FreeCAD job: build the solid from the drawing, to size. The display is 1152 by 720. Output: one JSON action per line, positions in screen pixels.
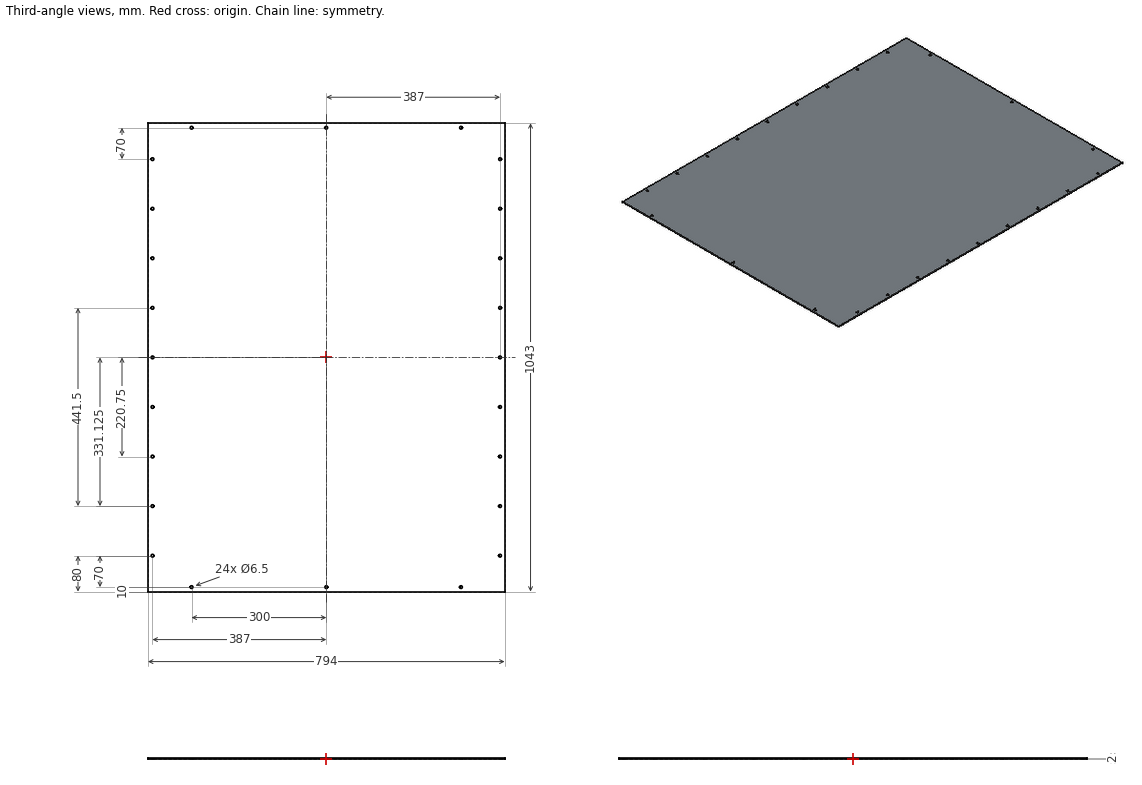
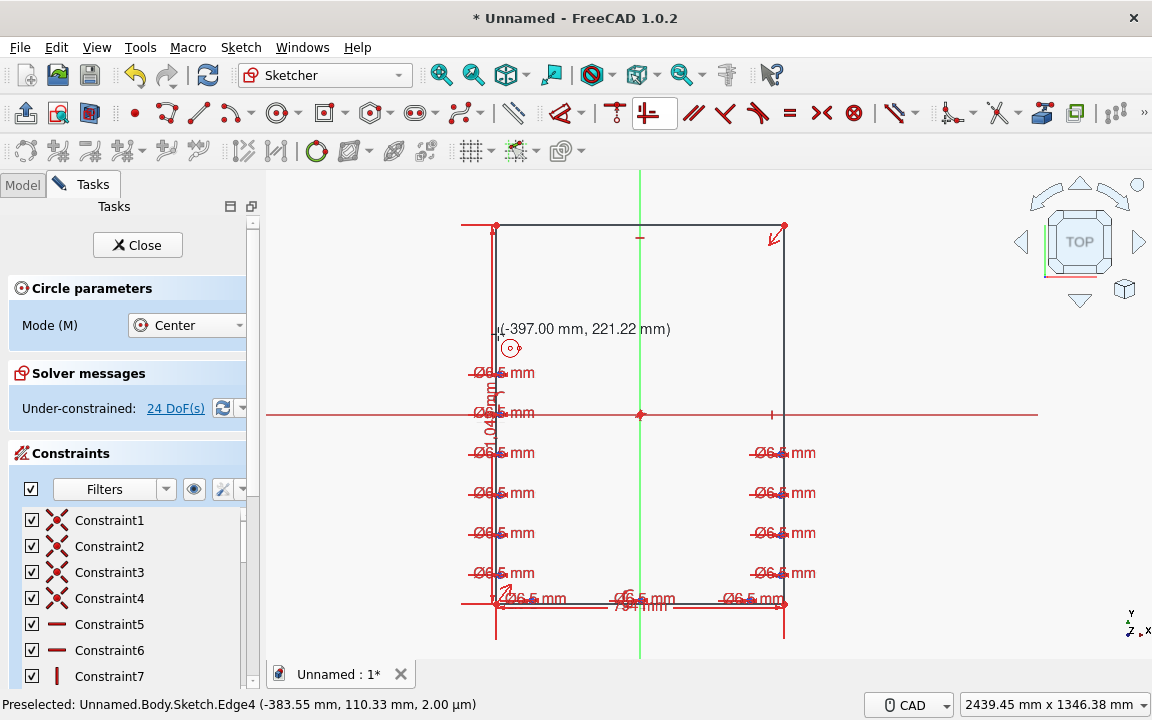
{"action": "scroll", "coordinate": [500, 335], "scroll_direction": "up", "scroll_amount": 8}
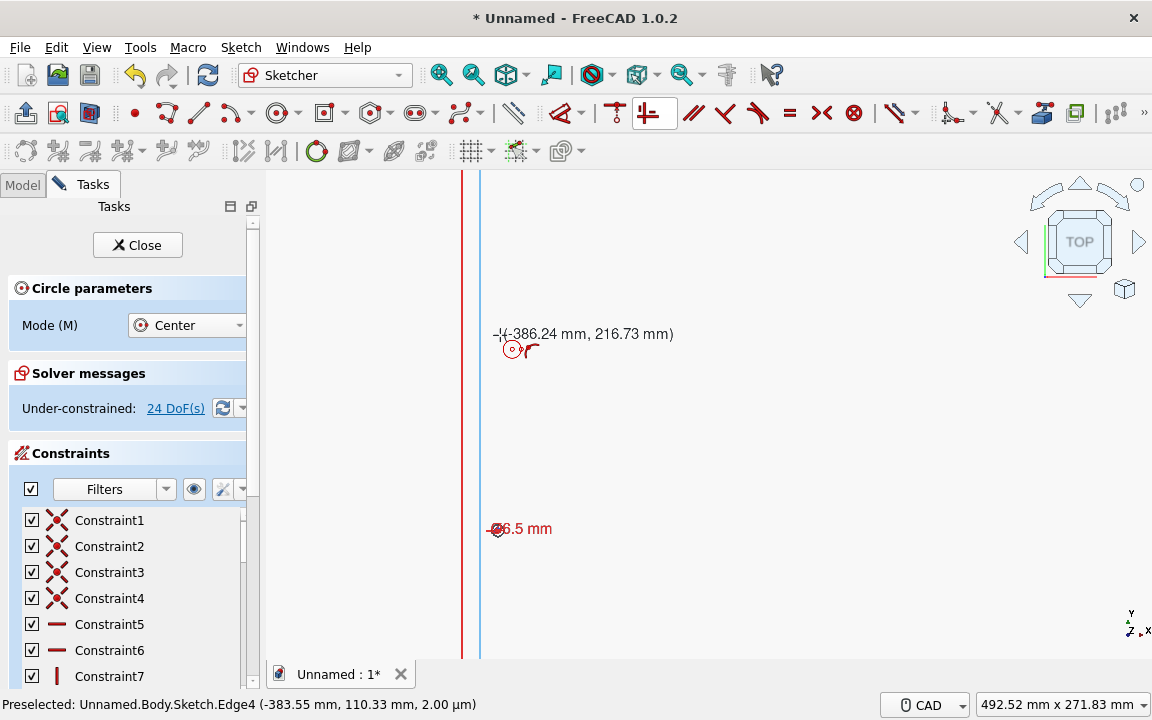
{"action": "left_click", "coordinate": [498, 331]}
{"action": "mouse_move", "coordinate": [502, 327]}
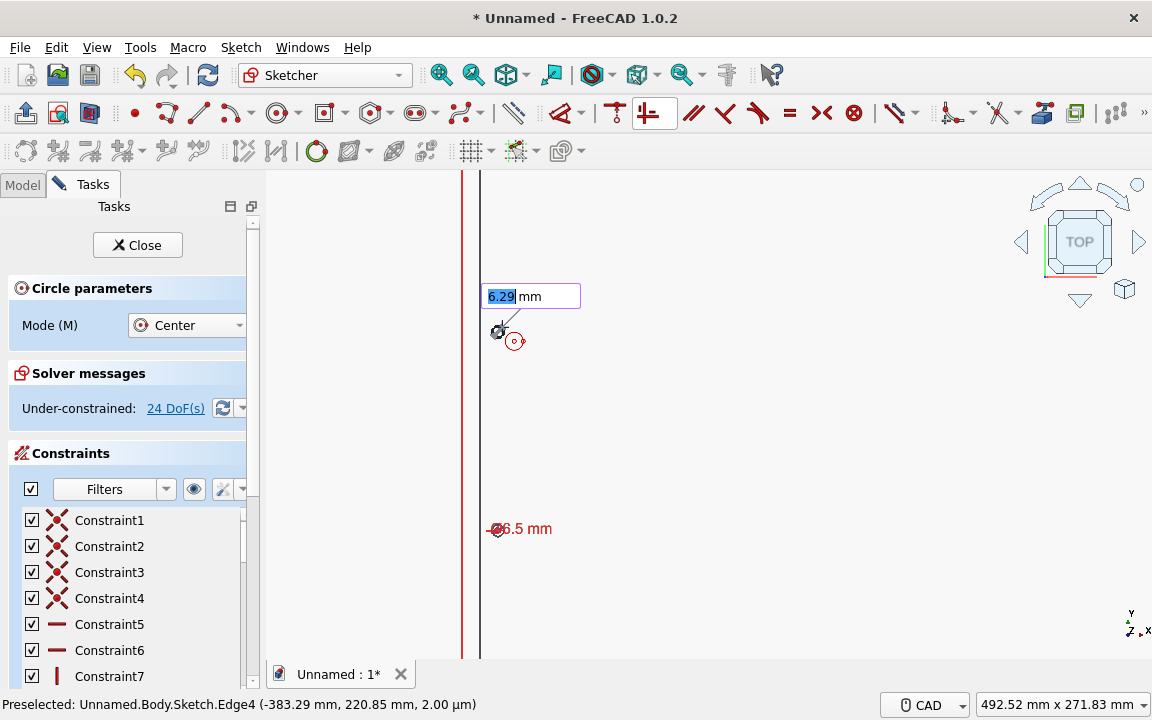
{"action": "type", "text": "6.5"}
{"action": "key", "text": "Return"}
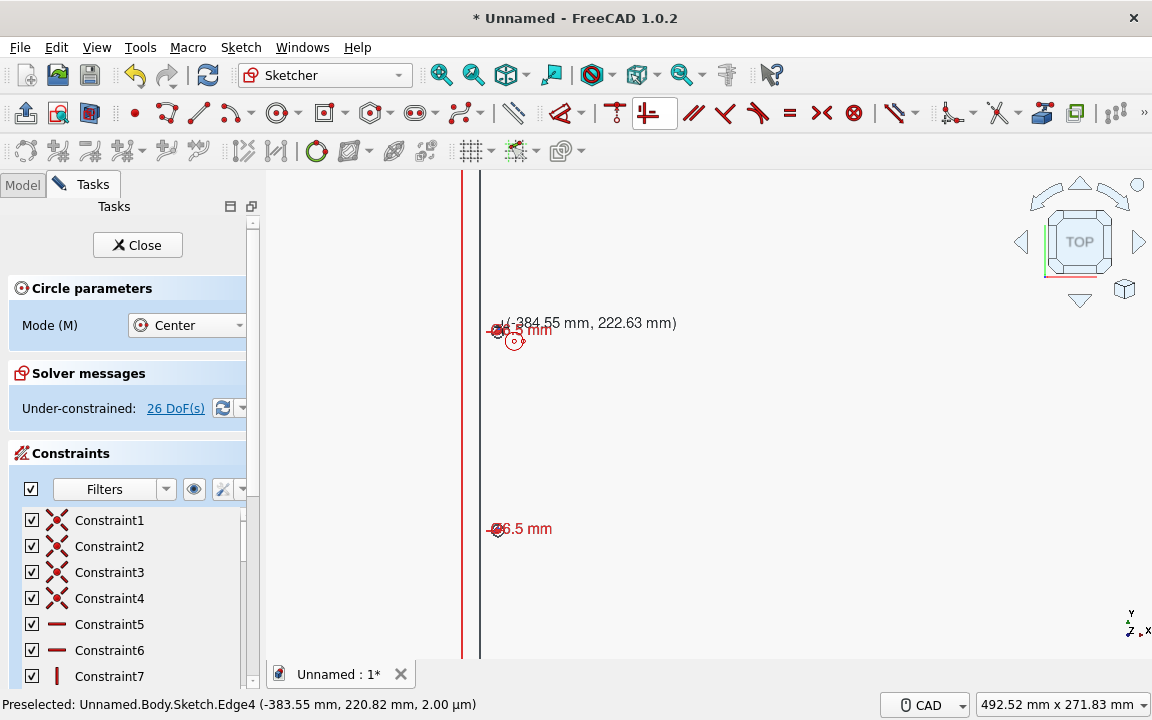
{"action": "scroll", "coordinate": [531, 352], "scroll_direction": "down", "scroll_amount": 9}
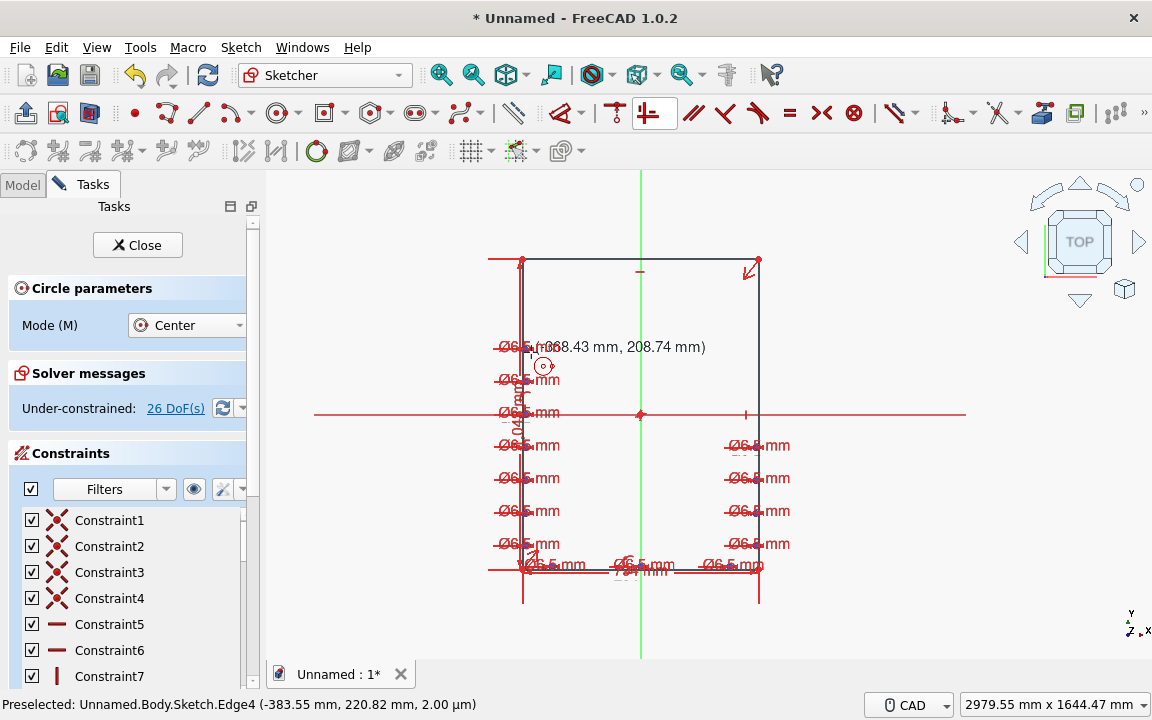
{"action": "scroll", "coordinate": [526, 316], "scroll_direction": "up", "scroll_amount": 16}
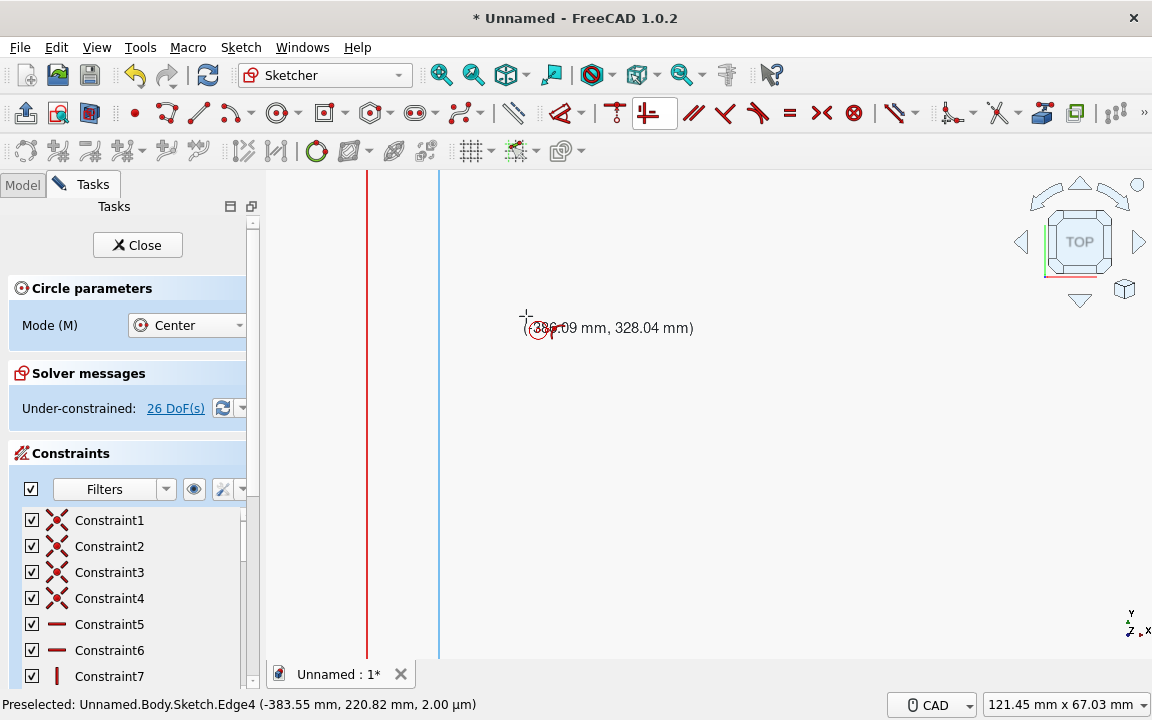
{"action": "scroll", "coordinate": [499, 293], "scroll_direction": "down", "scroll_amount": 15}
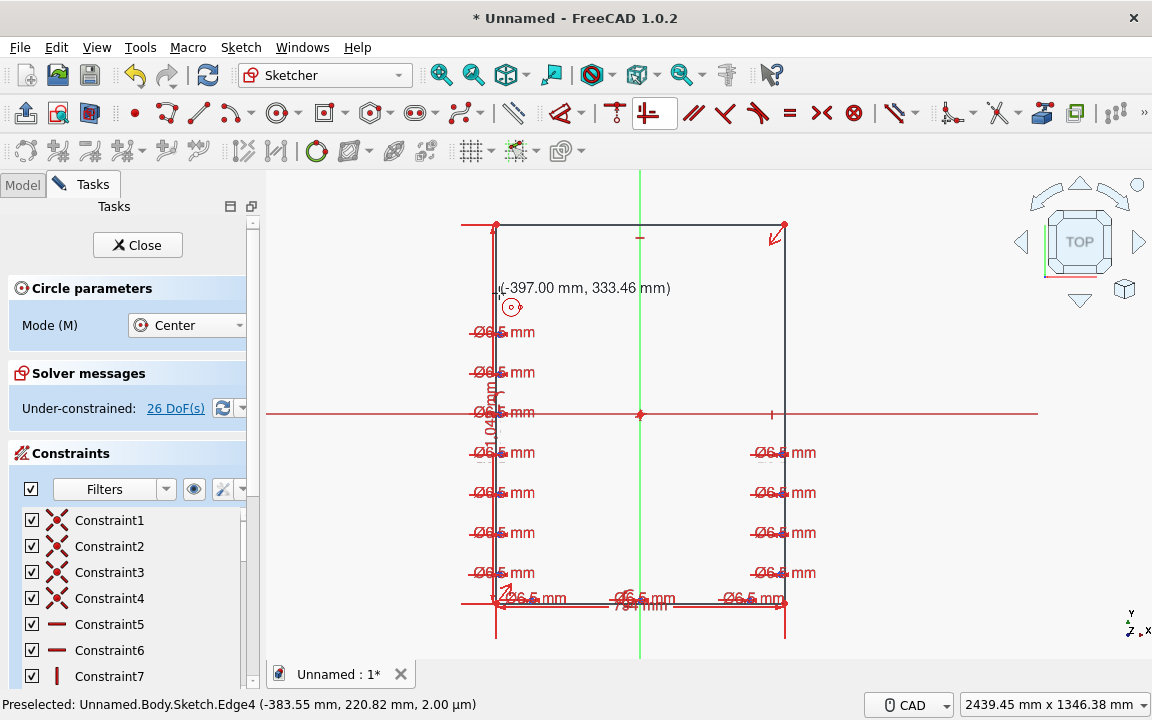
{"action": "scroll", "coordinate": [500, 294], "scroll_direction": "up", "scroll_amount": 8}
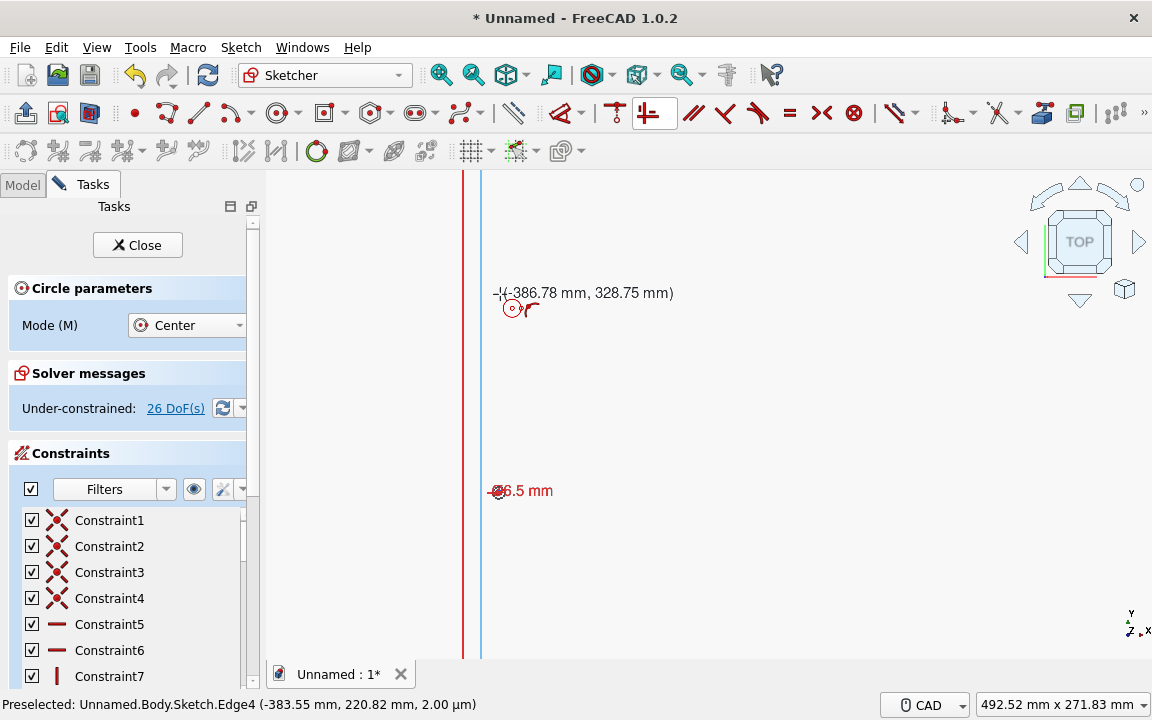
{"action": "left_click", "coordinate": [499, 294]}
{"action": "mouse_move", "coordinate": [503, 290]}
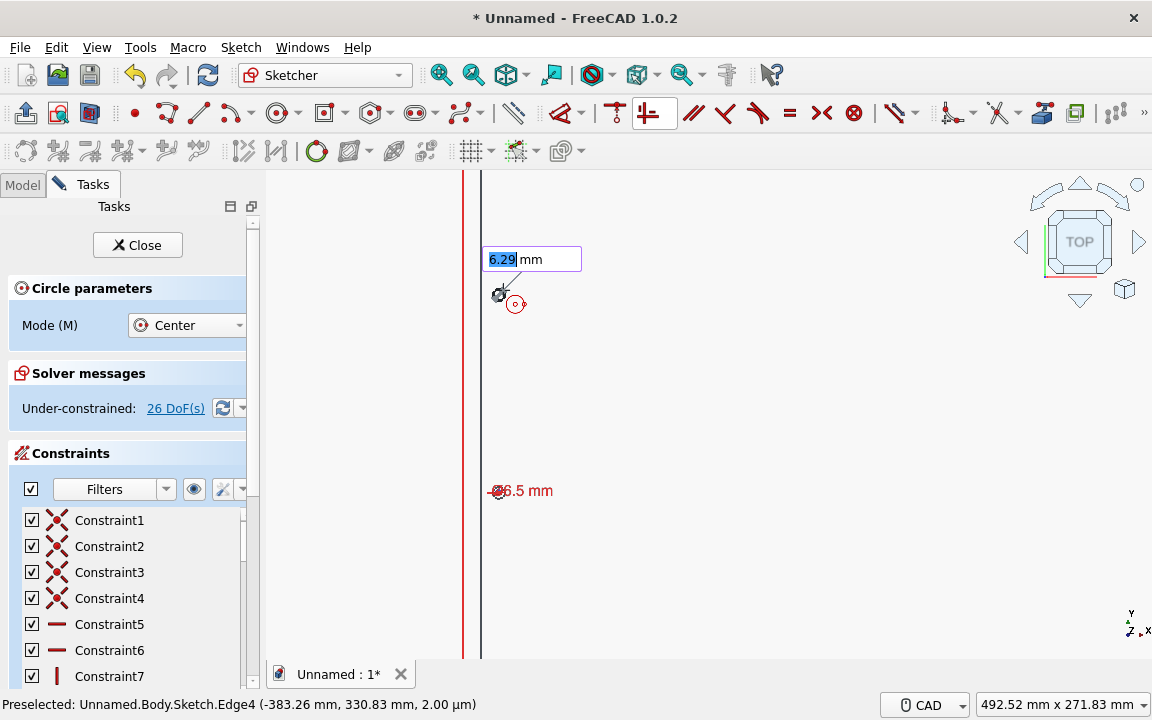
{"action": "type", "text": "6.5"}
{"action": "key", "text": "Return"}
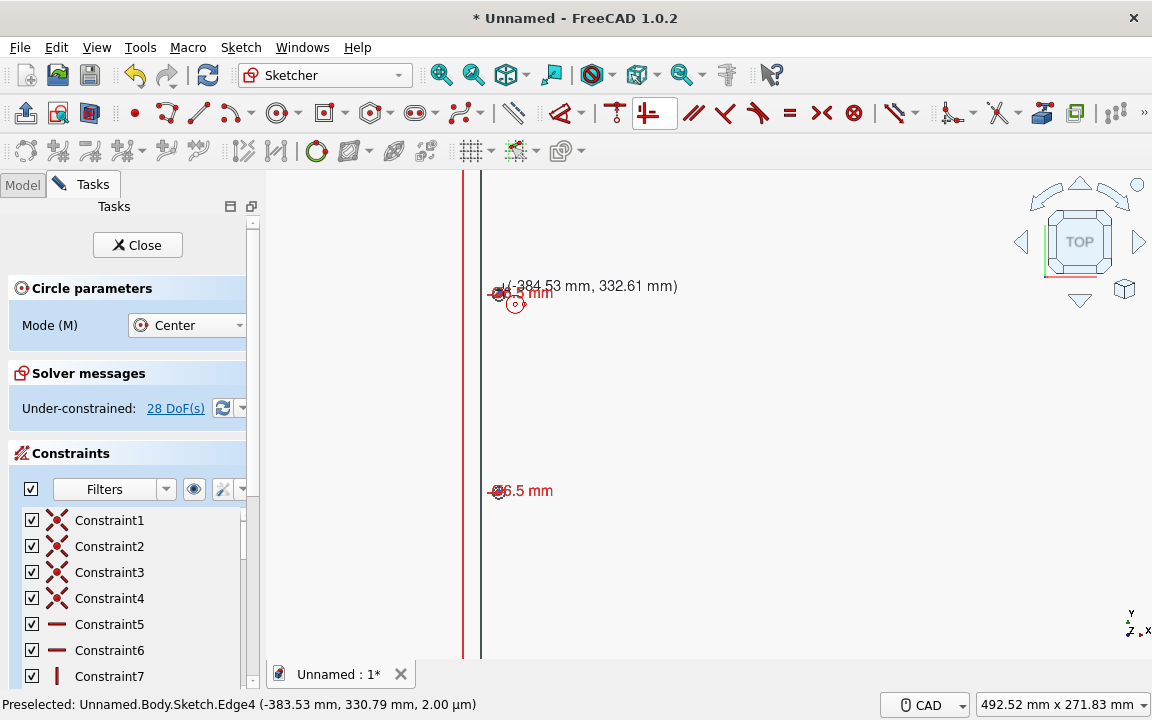
{"action": "scroll", "coordinate": [531, 320], "scroll_direction": "down", "scroll_amount": 9}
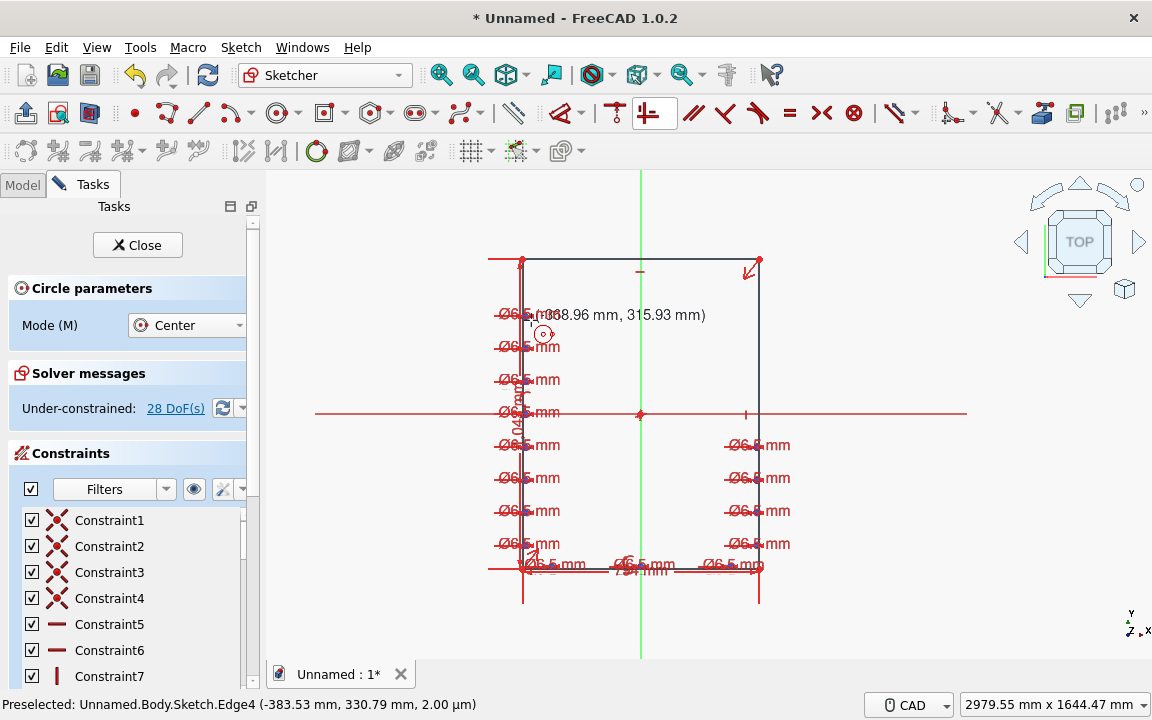
{"action": "scroll", "coordinate": [526, 283], "scroll_direction": "up", "scroll_amount": 16}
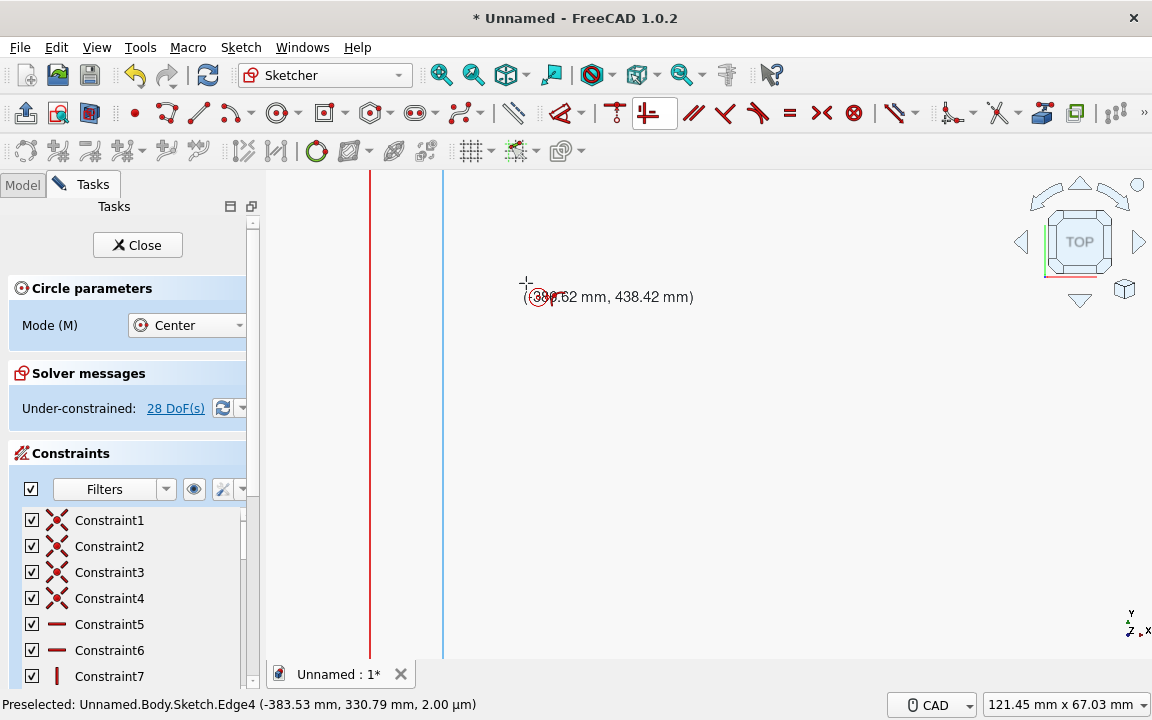
{"action": "scroll", "coordinate": [499, 253], "scroll_direction": "down", "scroll_amount": 15}